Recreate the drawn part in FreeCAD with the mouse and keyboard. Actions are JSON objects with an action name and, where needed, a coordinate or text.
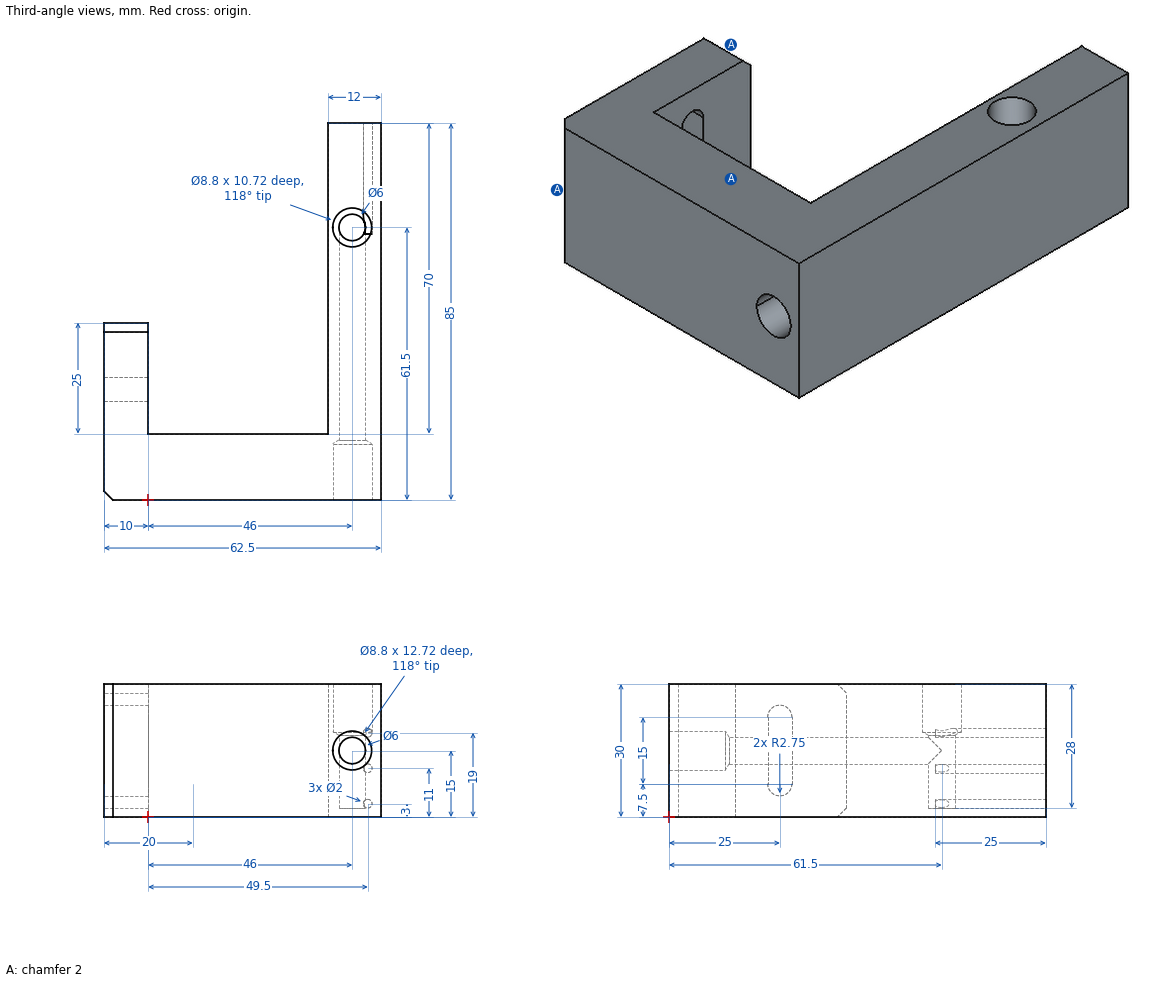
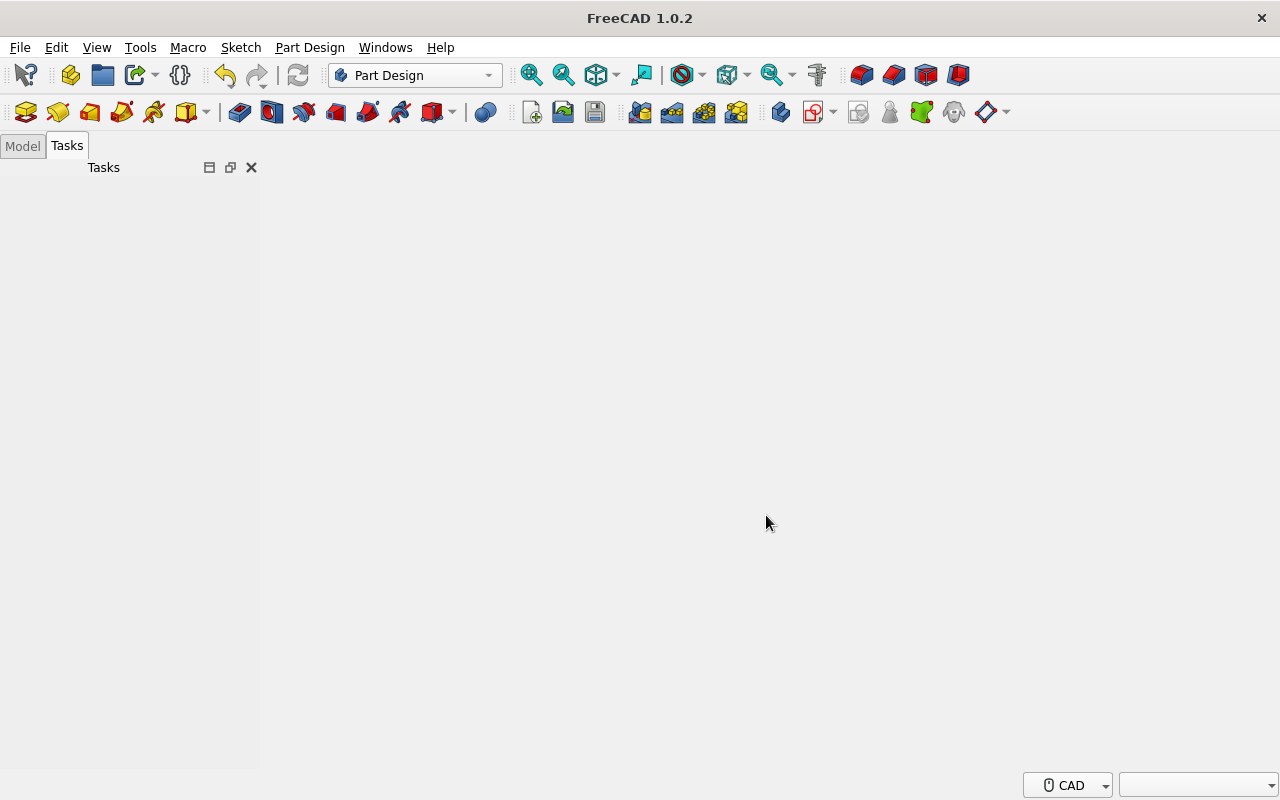
{"action": "key", "text": "ctrl+n"}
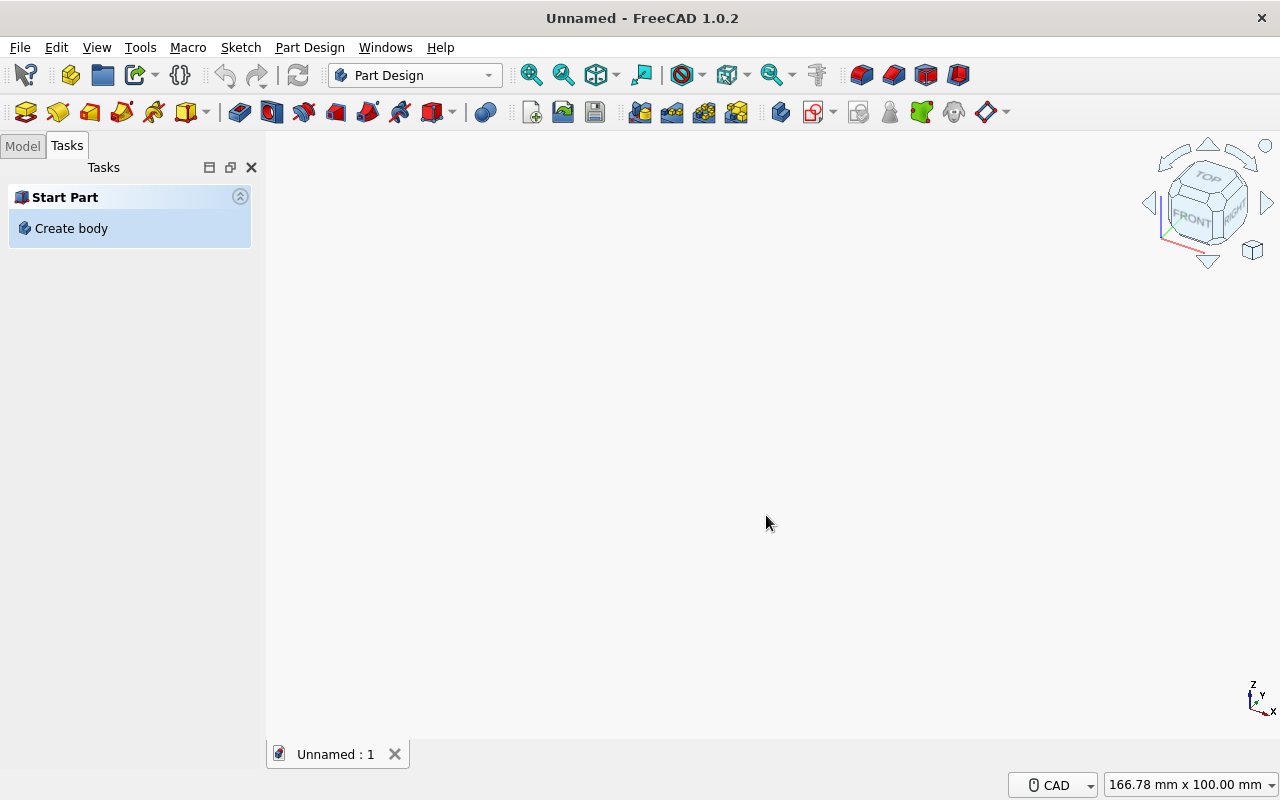
{"action": "left_click", "coordinate": [814, 112]}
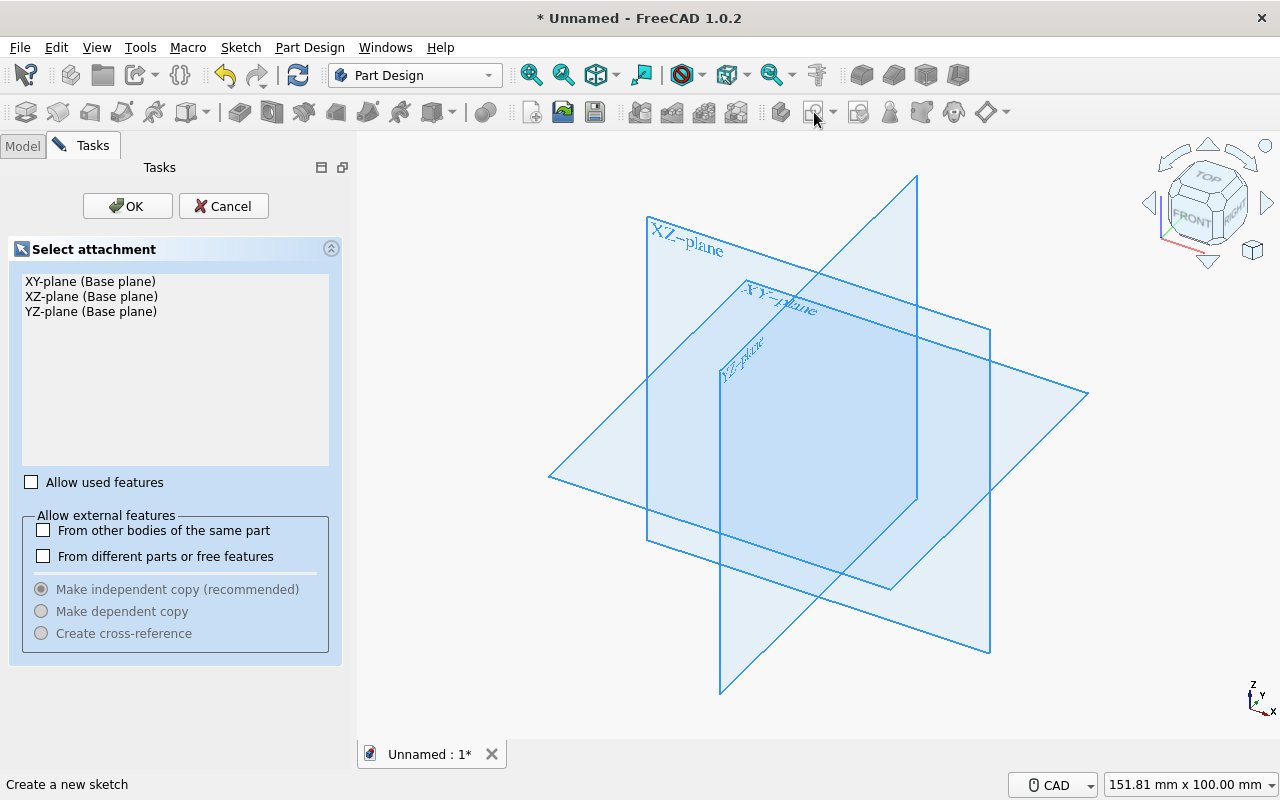
{"action": "left_click", "coordinate": [82, 282]}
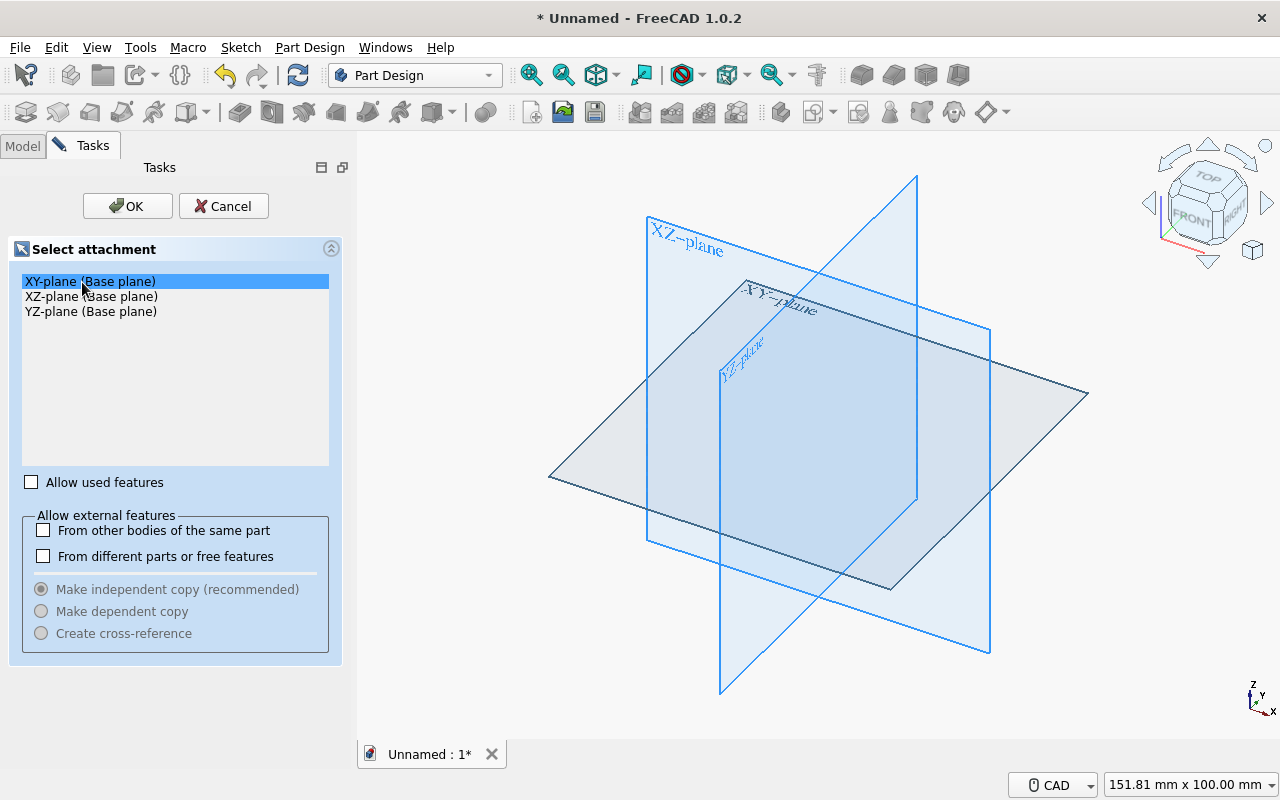
{"action": "left_click", "coordinate": [128, 206]}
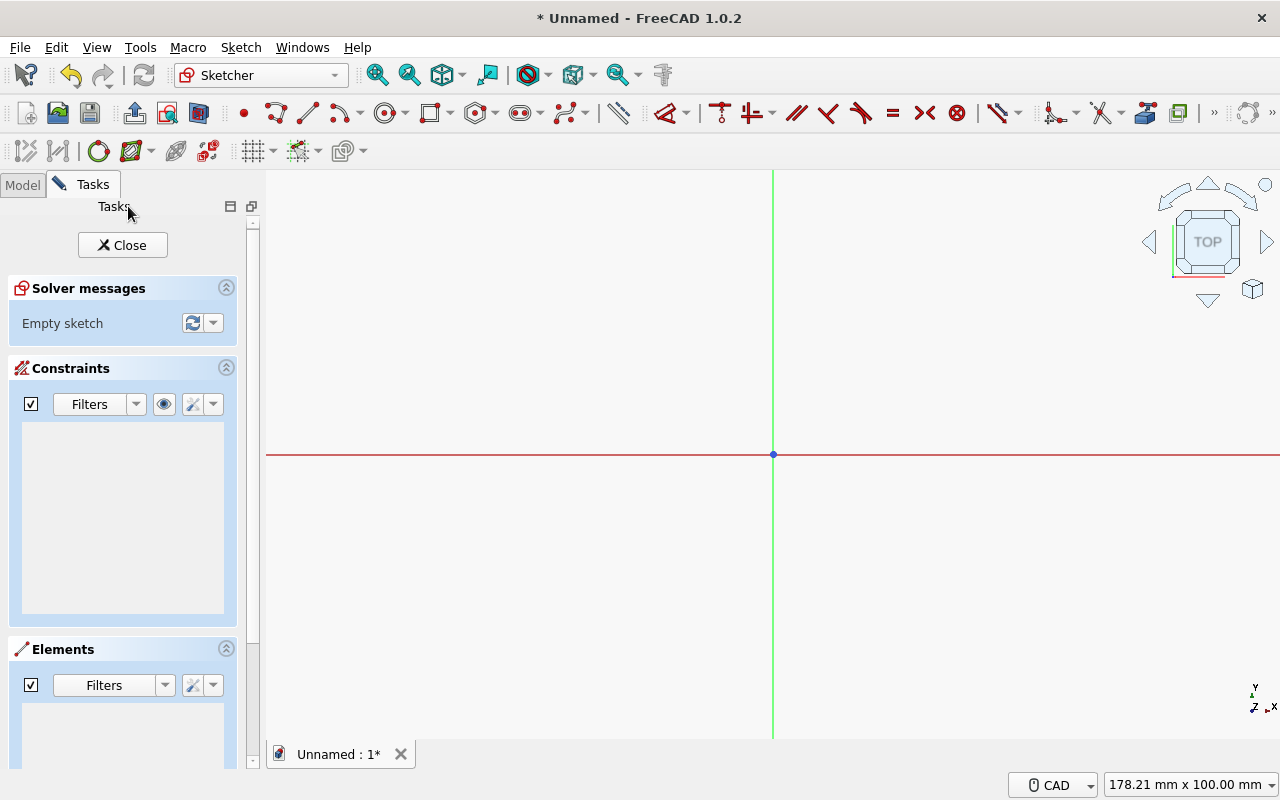
{"action": "scroll", "coordinate": [474, 711], "scroll_direction": "down", "scroll_amount": 3}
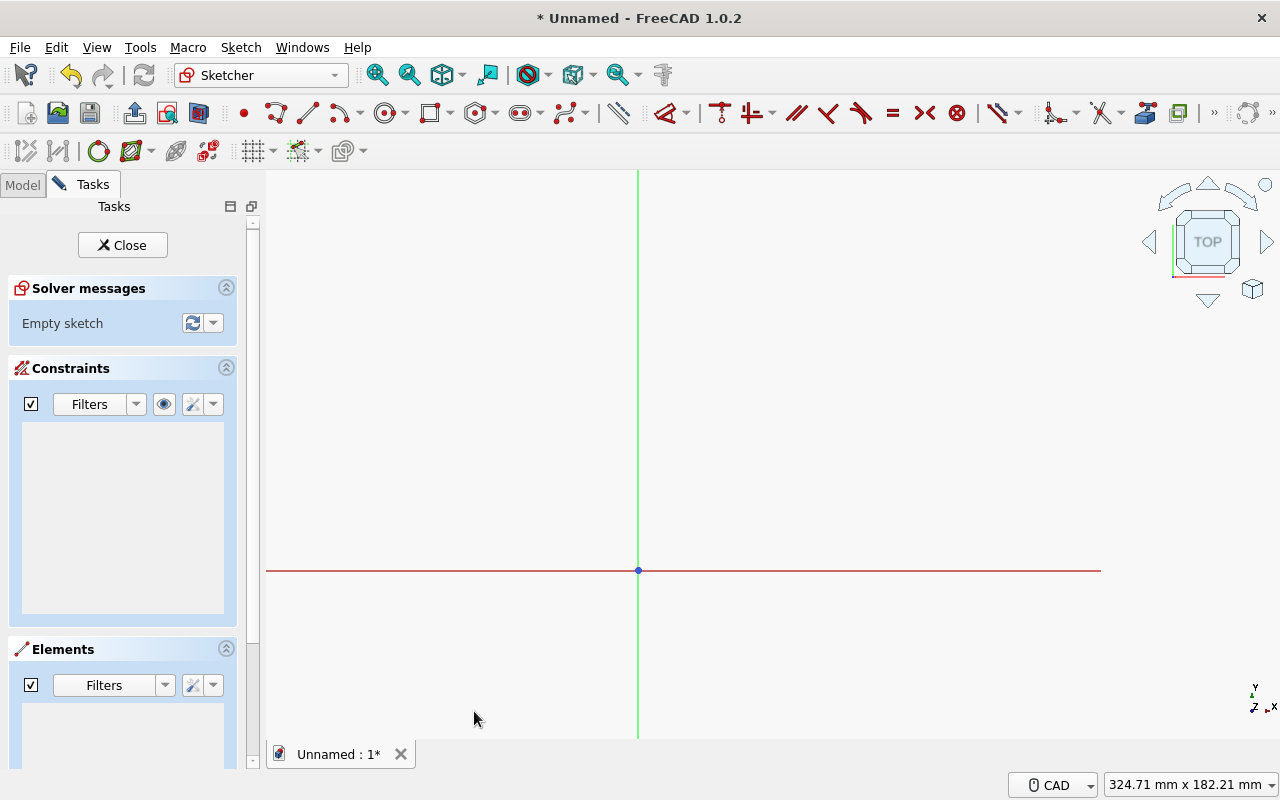
{"action": "scroll", "coordinate": [705, 404], "scroll_direction": "up", "scroll_amount": 2}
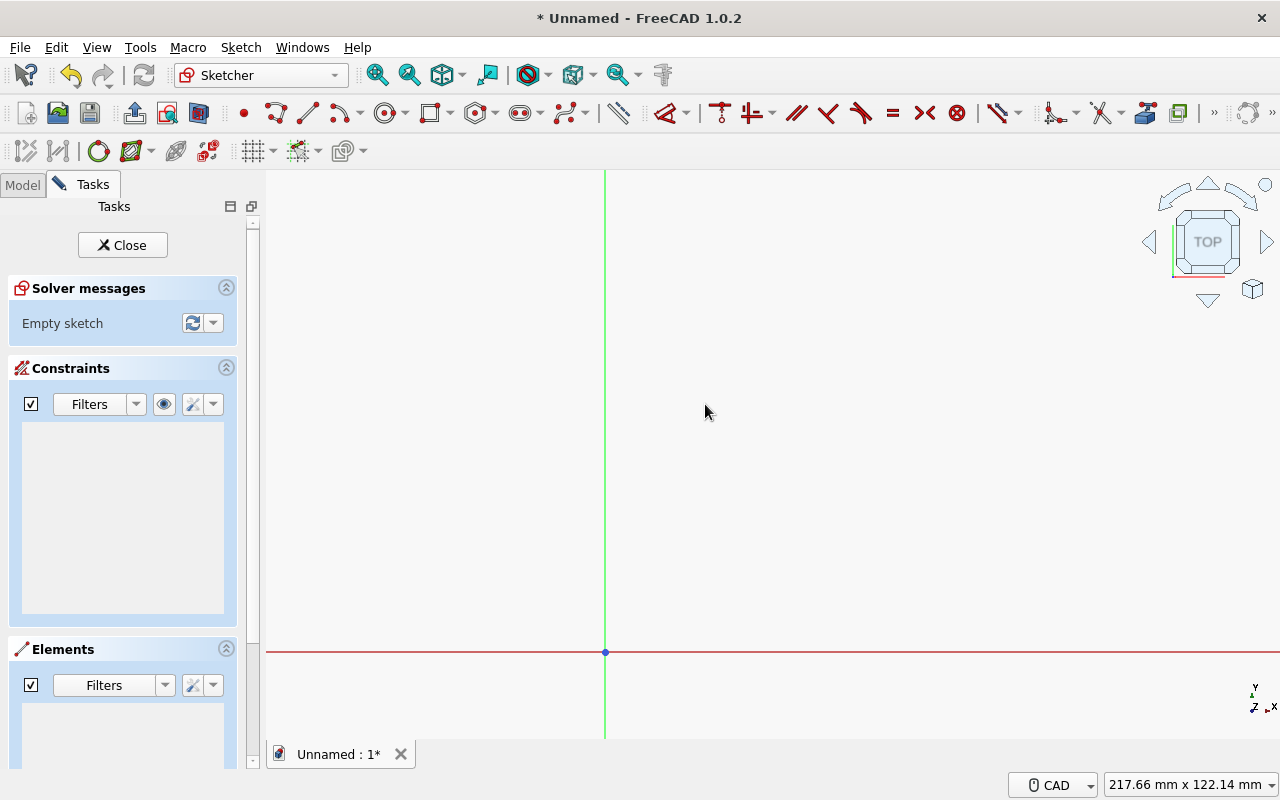
{"action": "key", "text": "g m"}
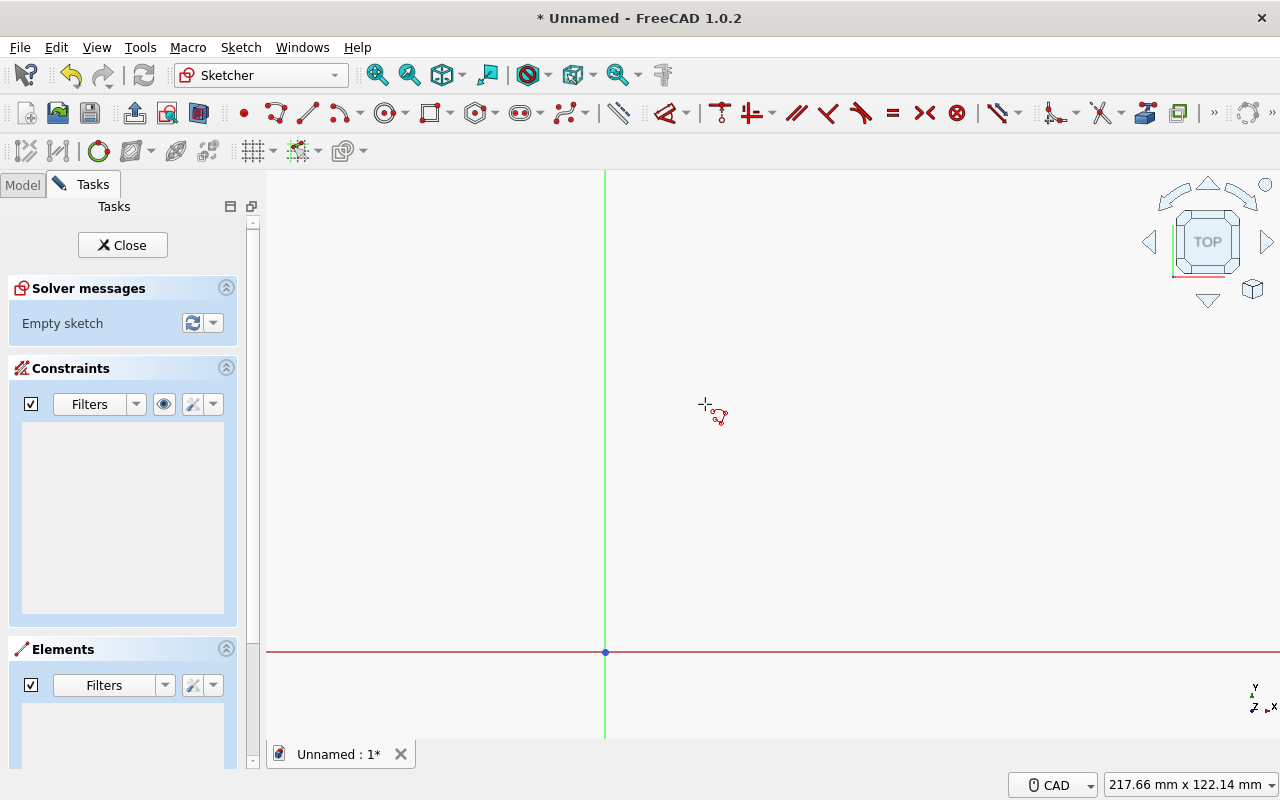
{"action": "left_click", "coordinate": [559, 652]}
{"action": "left_click", "coordinate": [850, 643]}
{"action": "left_click", "coordinate": [850, 256]}
{"action": "left_click", "coordinate": [794, 256]}
{"action": "left_click", "coordinate": [794, 583]}
{"action": "left_click", "coordinate": [605, 583]}
{"action": "left_click", "coordinate": [614, 466]}
{"action": "left_click", "coordinate": [559, 466]}
{"action": "left_click", "coordinate": [559, 652]}
{"action": "key", "text": "Escape"}
{"action": "key", "text": "Escape"}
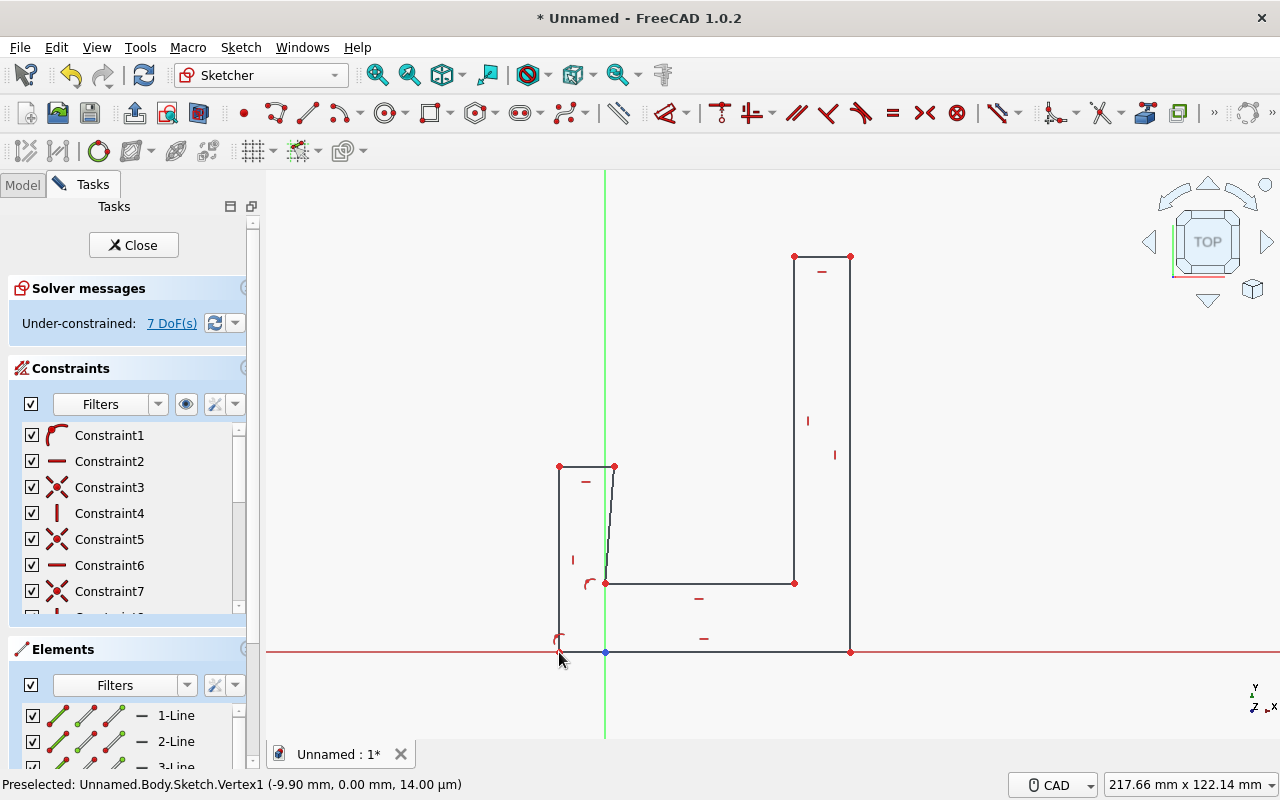
{"action": "left_click", "coordinate": [608, 549]}